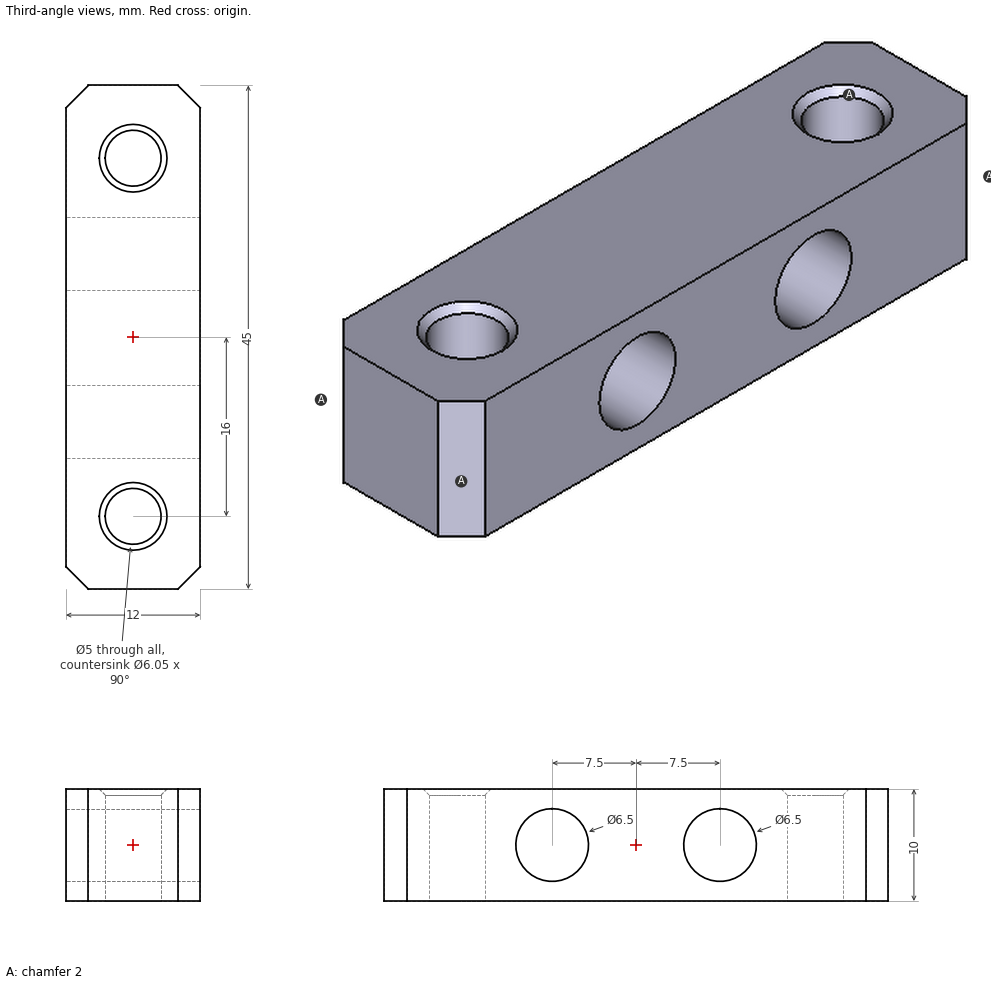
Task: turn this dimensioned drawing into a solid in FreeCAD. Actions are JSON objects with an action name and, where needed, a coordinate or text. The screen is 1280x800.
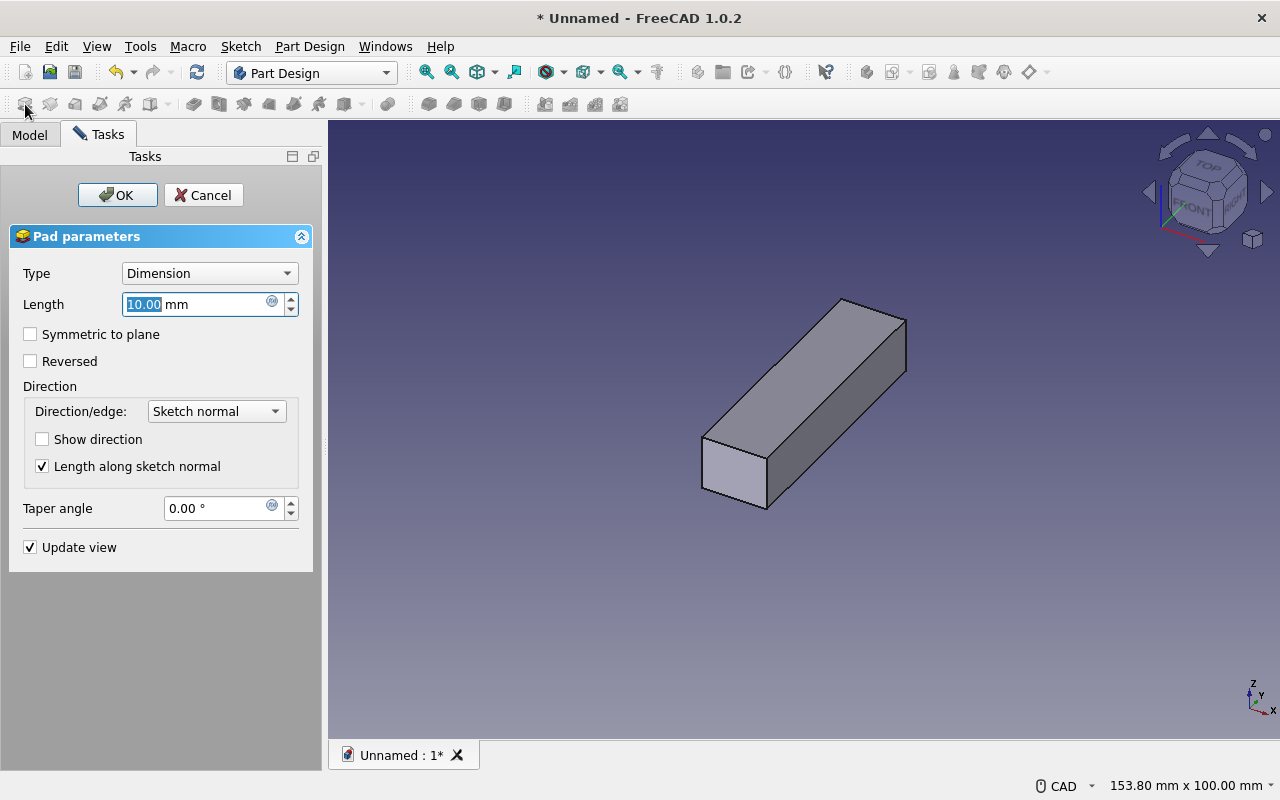
{"action": "type", "text": "10"}
{"action": "key", "text": "Tab"}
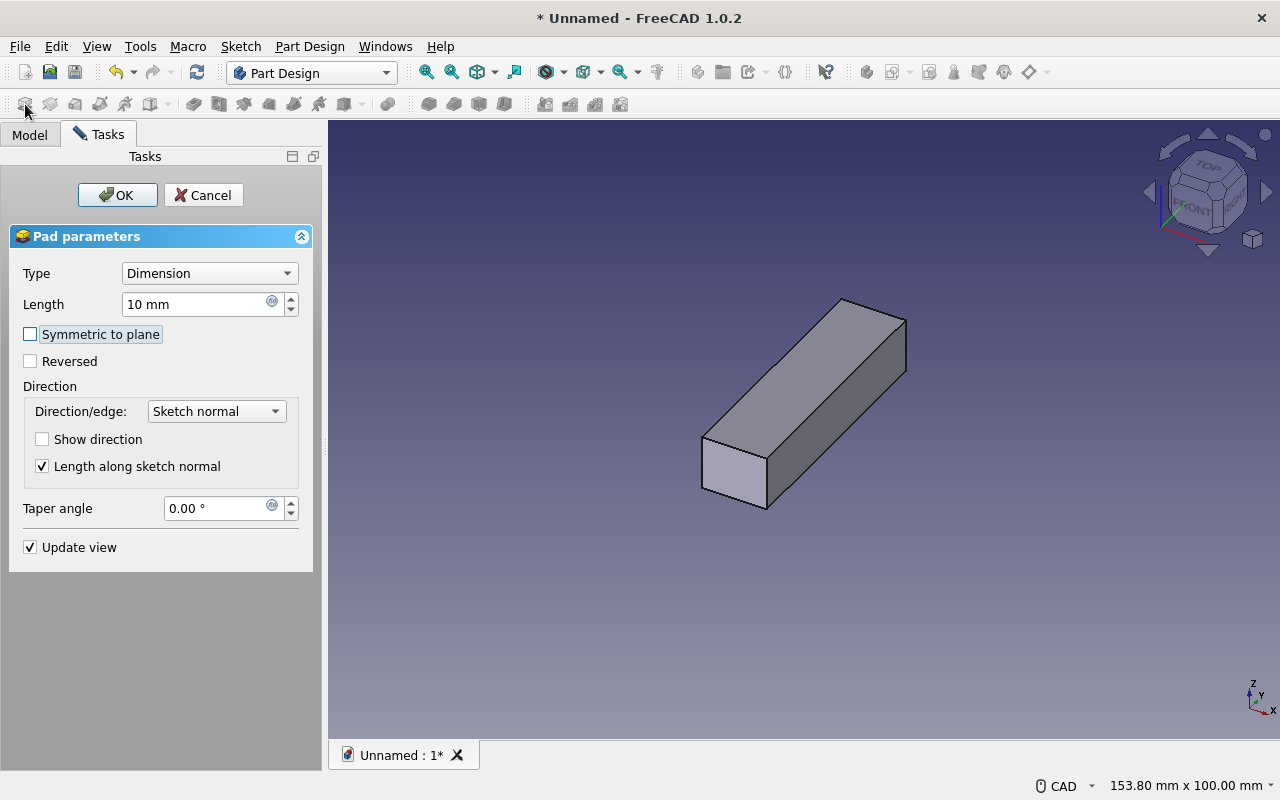
{"action": "left_click", "coordinate": [31, 334]}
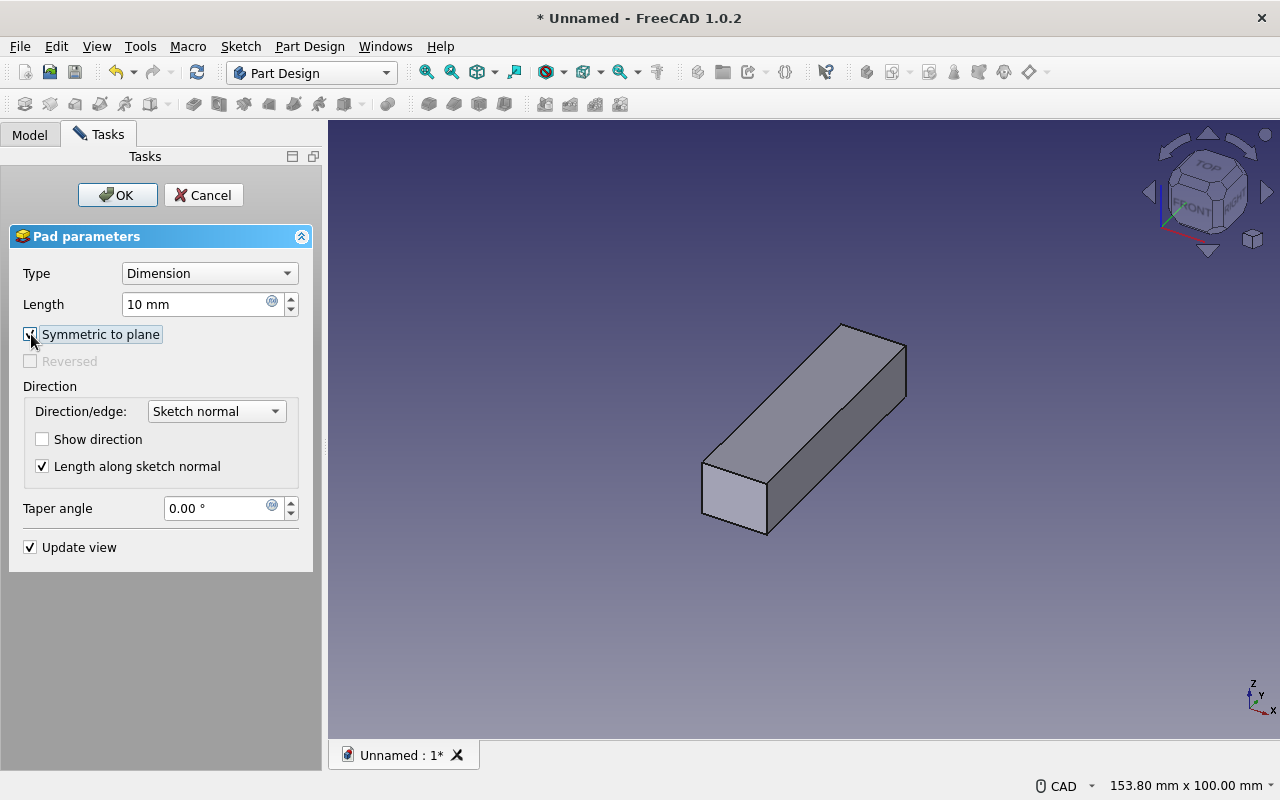
{"action": "left_click", "coordinate": [118, 195]}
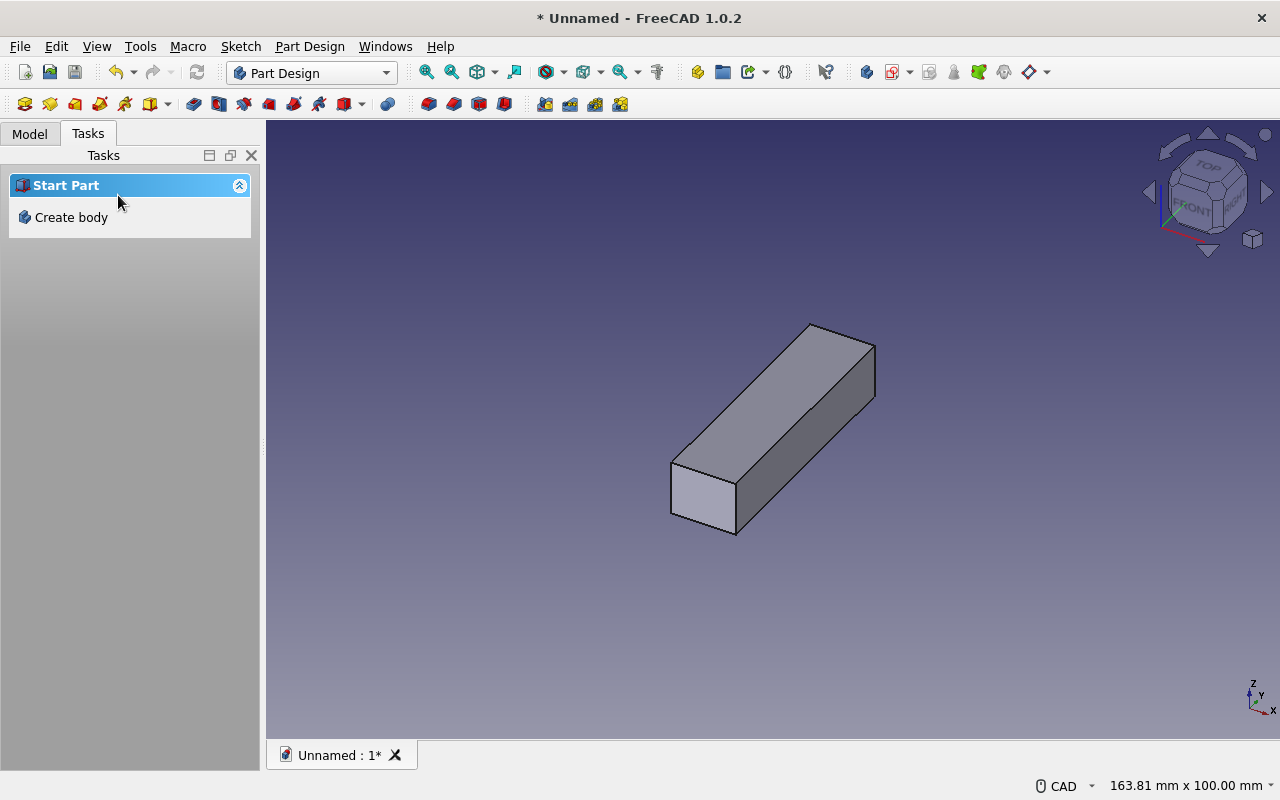
{"action": "left_click", "coordinate": [427, 72]}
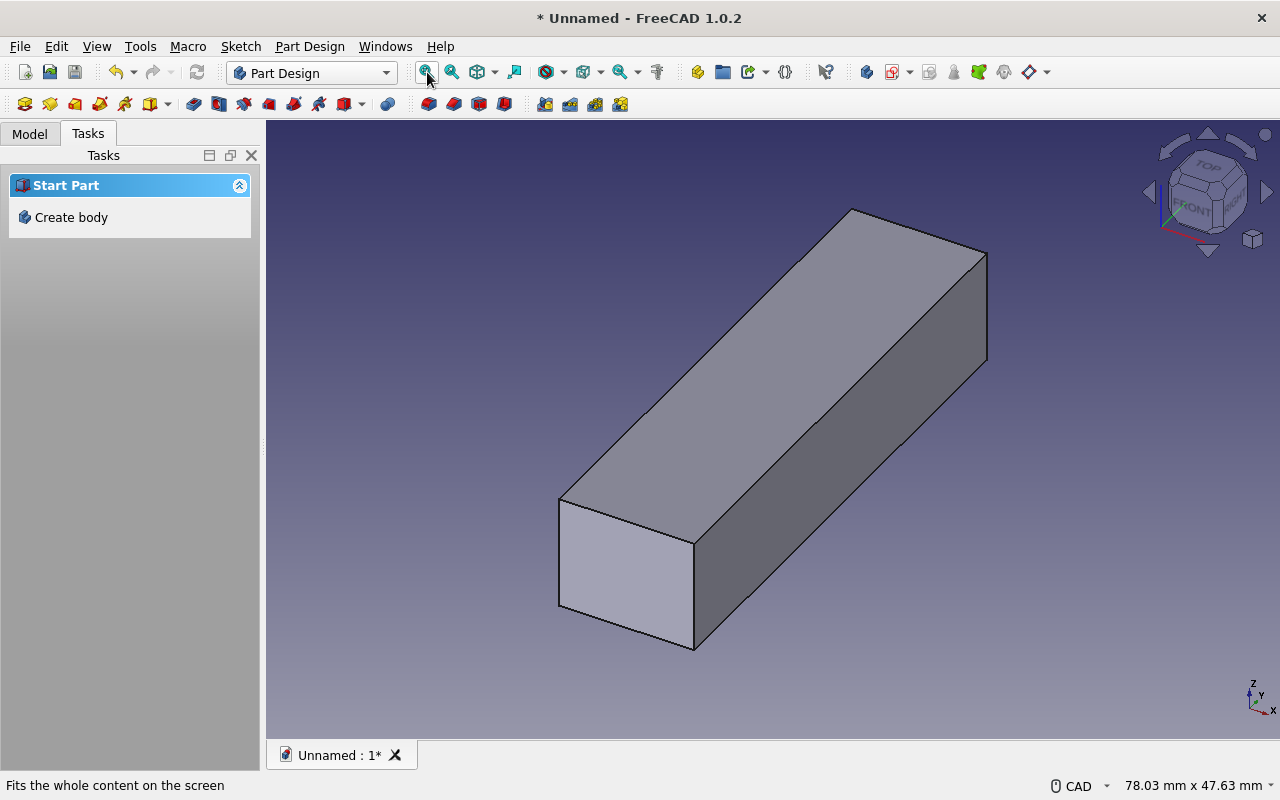
{"action": "left_click", "coordinate": [857, 292]}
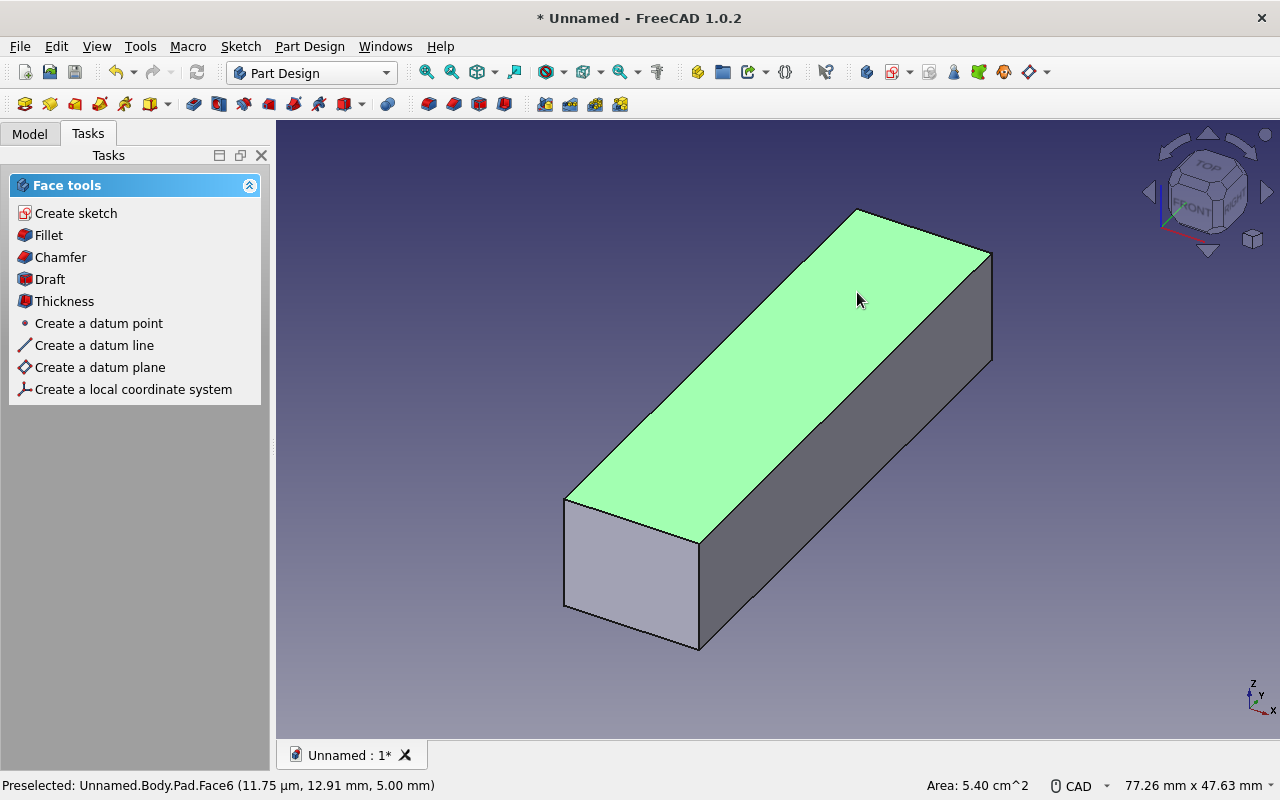
{"action": "left_click", "coordinate": [892, 72]}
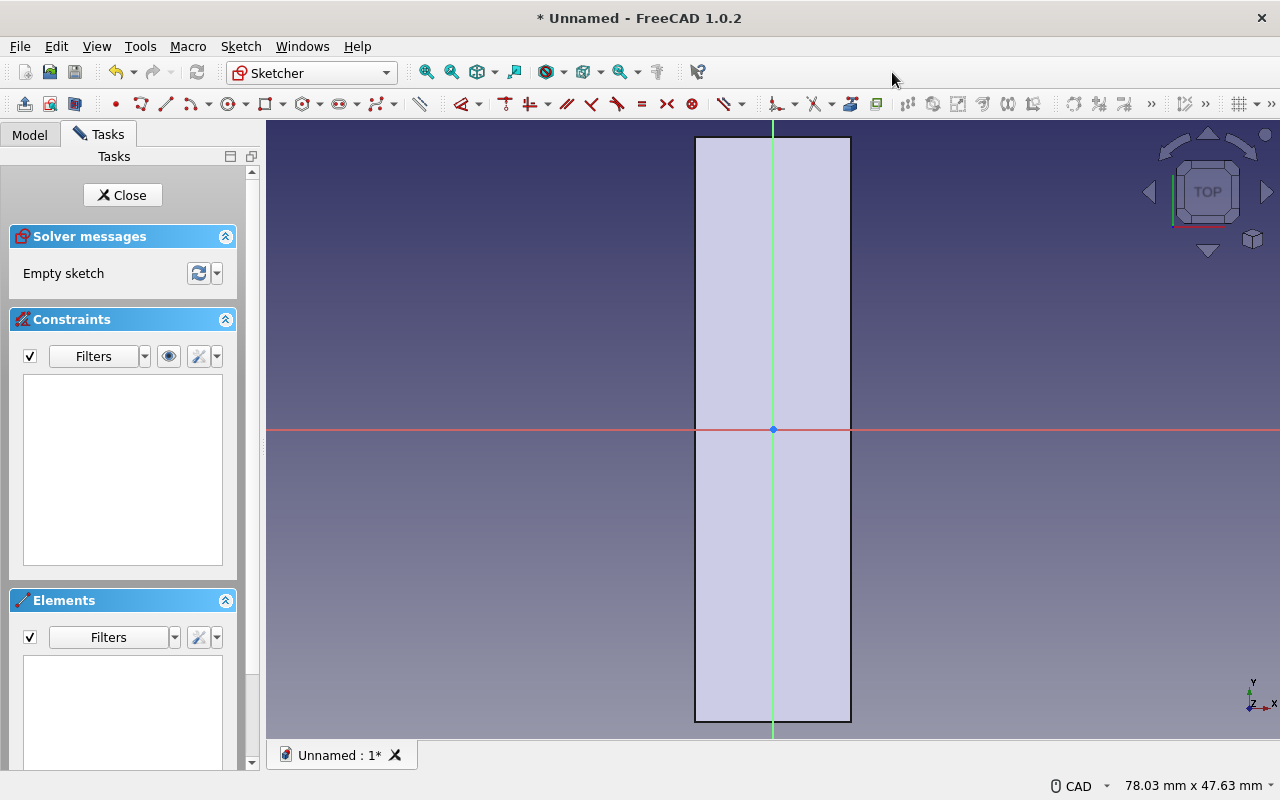
{"action": "scroll", "coordinate": [787, 679], "scroll_direction": "up", "scroll_amount": 9}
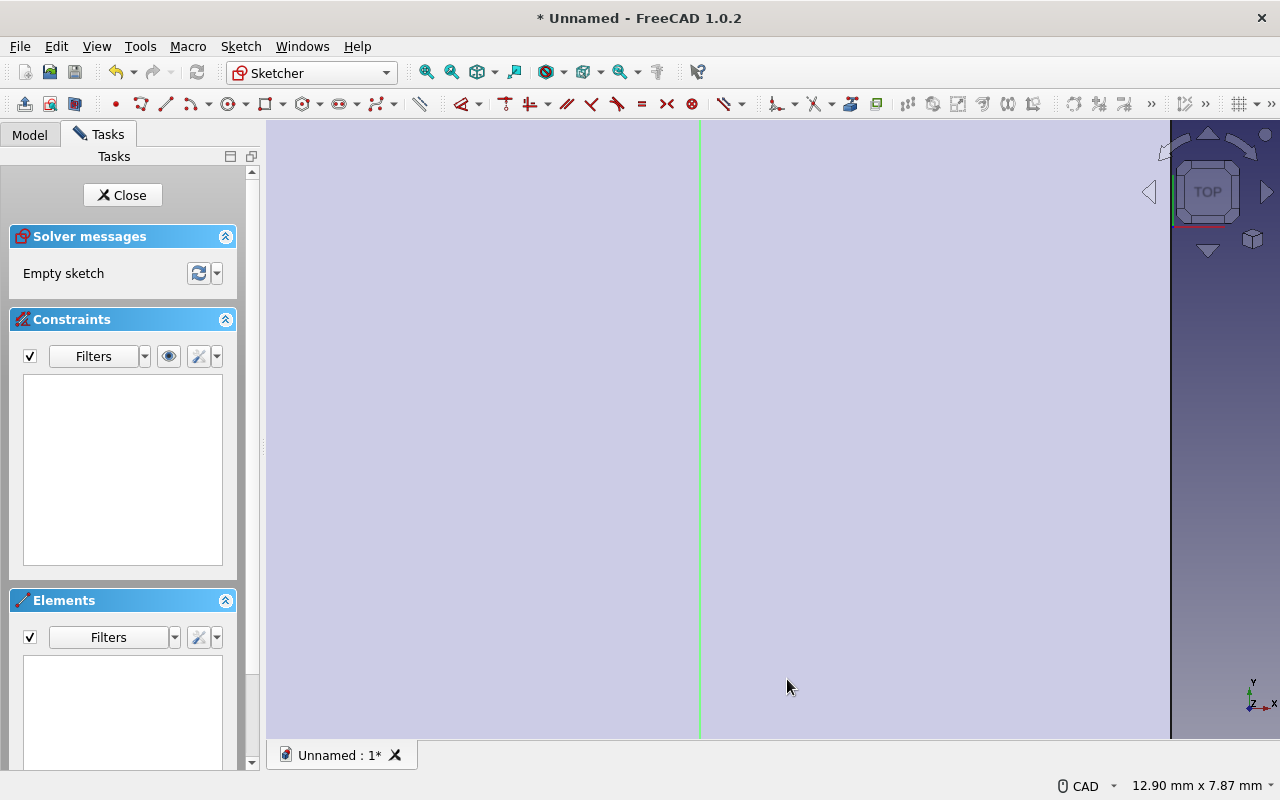
{"action": "left_click", "coordinate": [228, 104]}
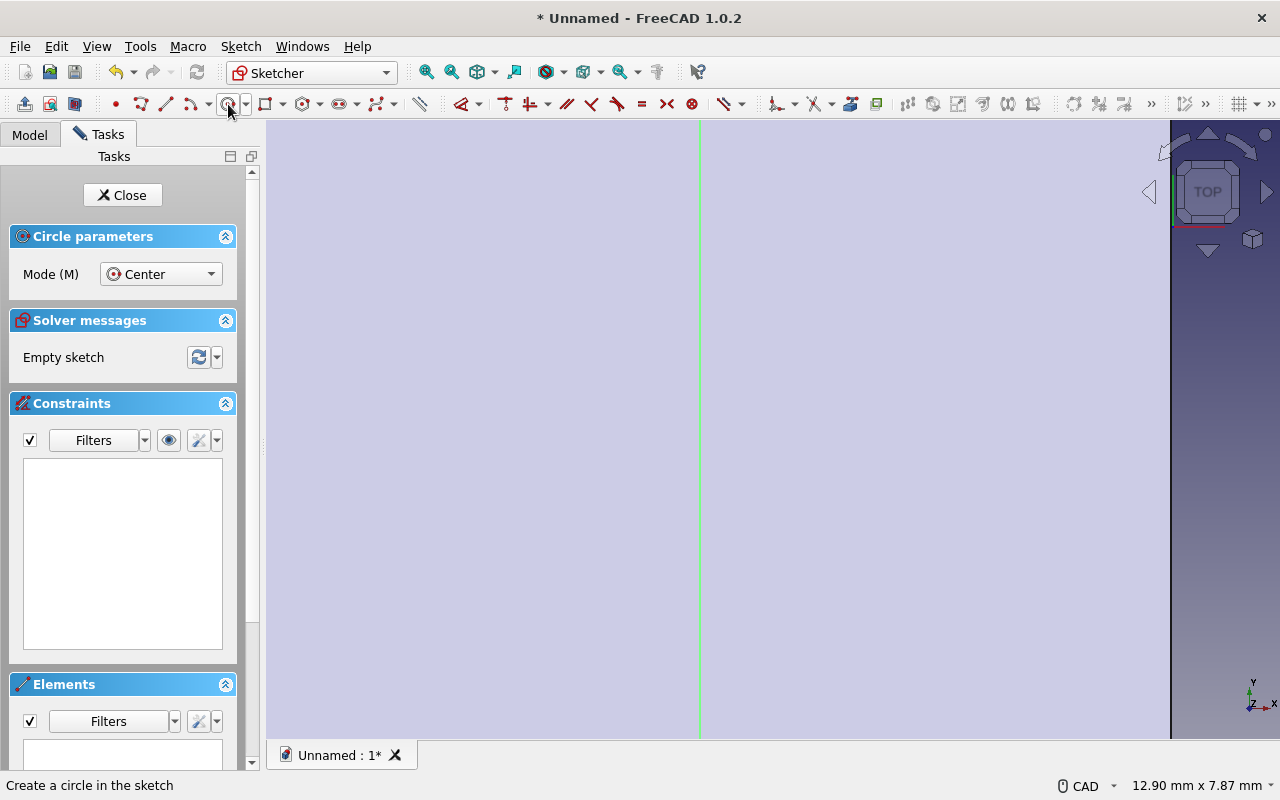
{"action": "left_click", "coordinate": [700, 423]}
{"action": "mouse_move", "coordinate": [839, 284]}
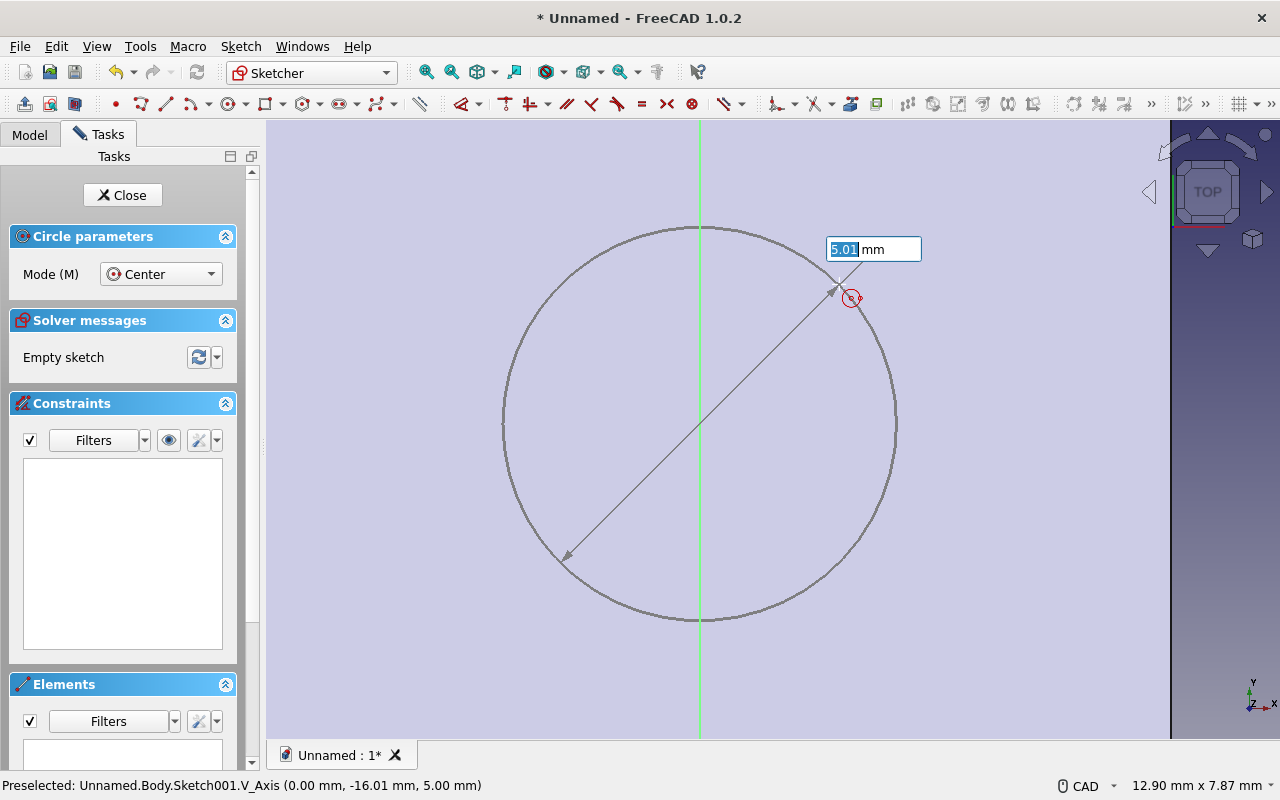
{"action": "type", "text": "5"}
{"action": "key", "text": "Return"}
{"action": "key", "text": "Escape"}